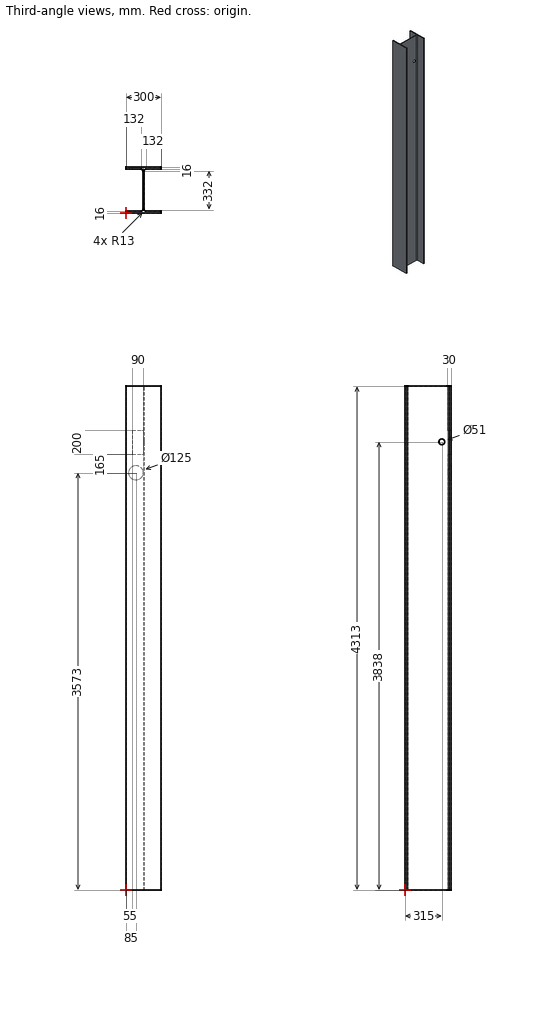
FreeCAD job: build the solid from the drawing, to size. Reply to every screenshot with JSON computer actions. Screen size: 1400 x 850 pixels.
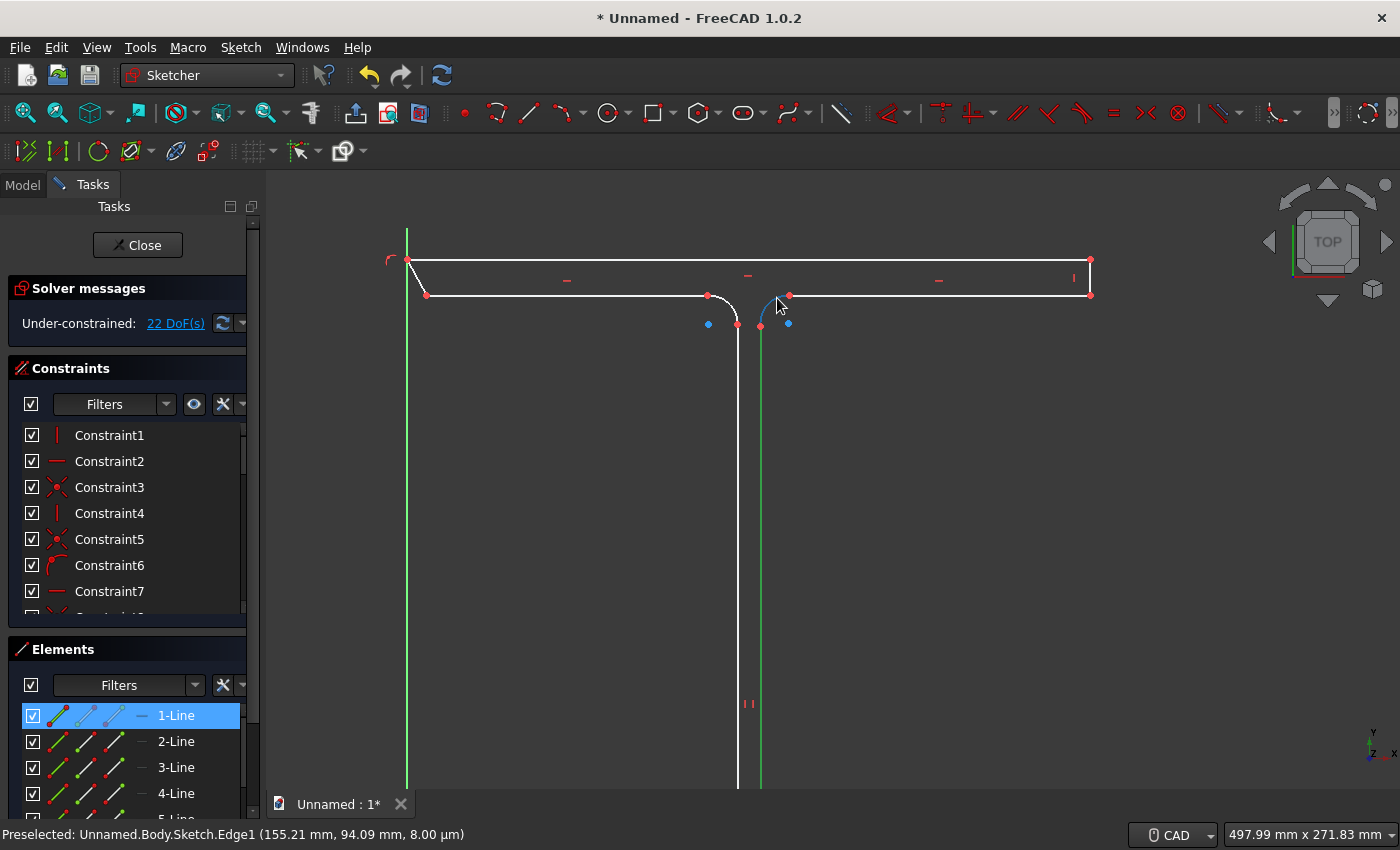
{"action": "left_click", "coordinate": [776, 299]}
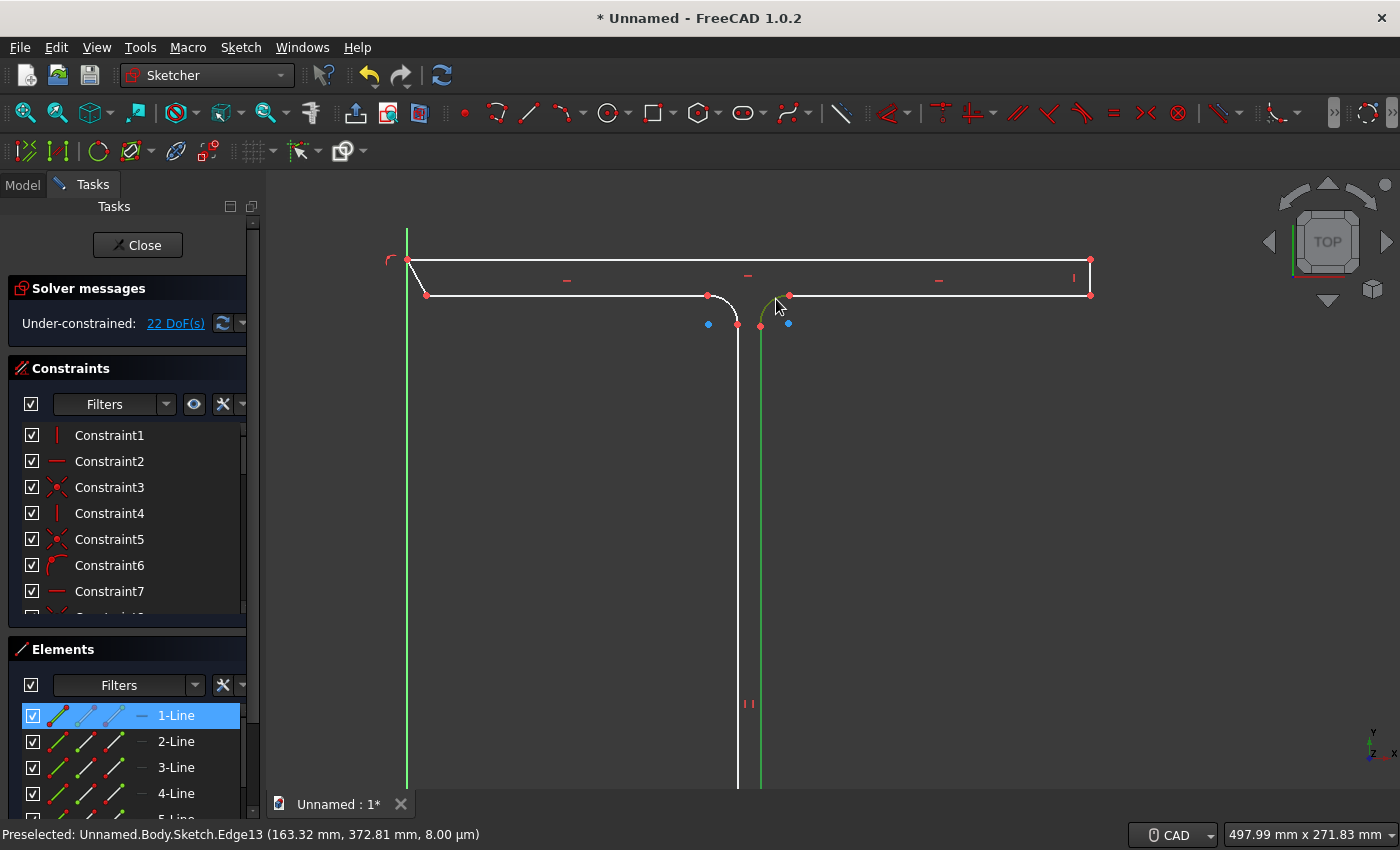
{"action": "key", "text": "t"}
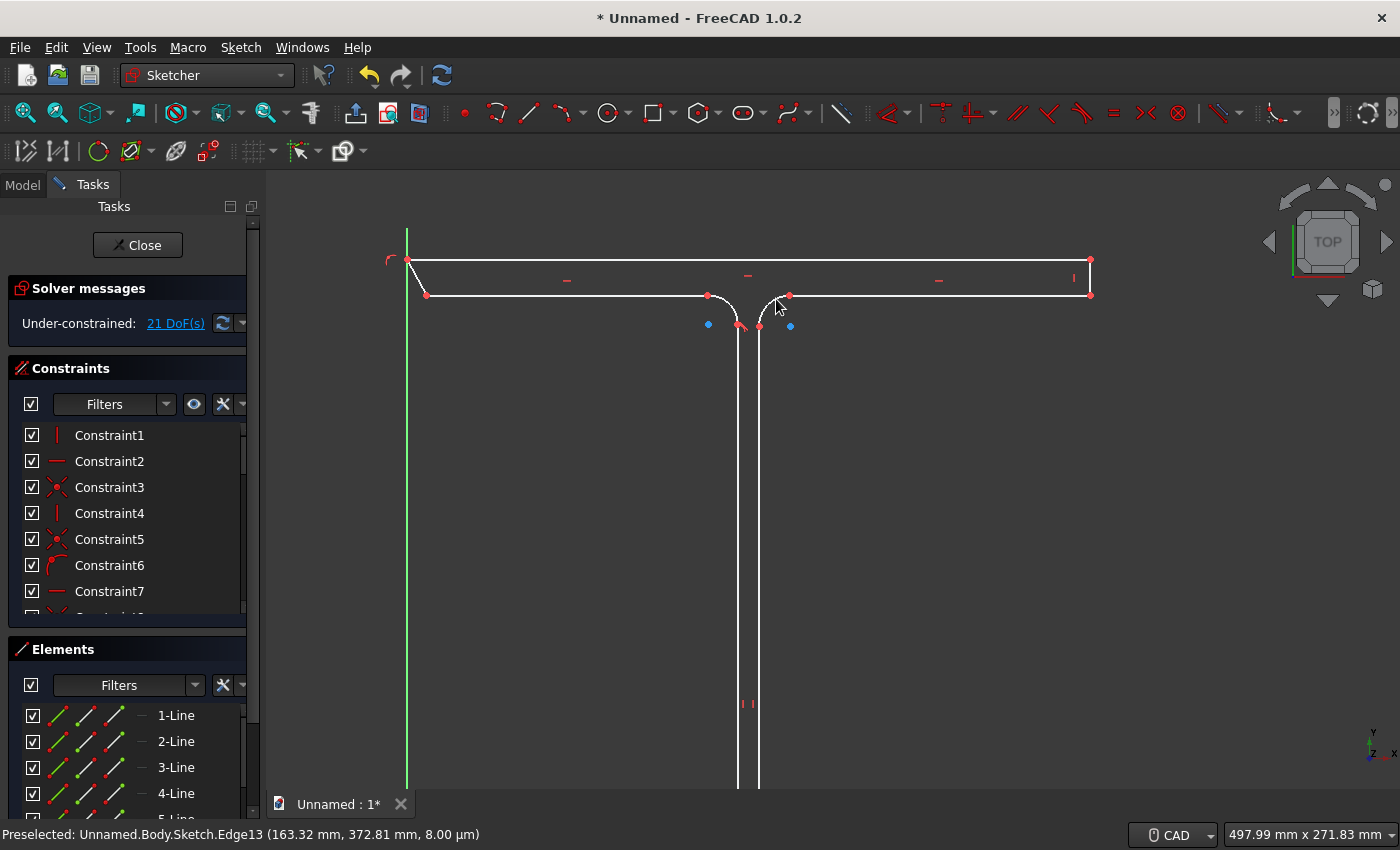
{"action": "left_click", "coordinate": [759, 553]}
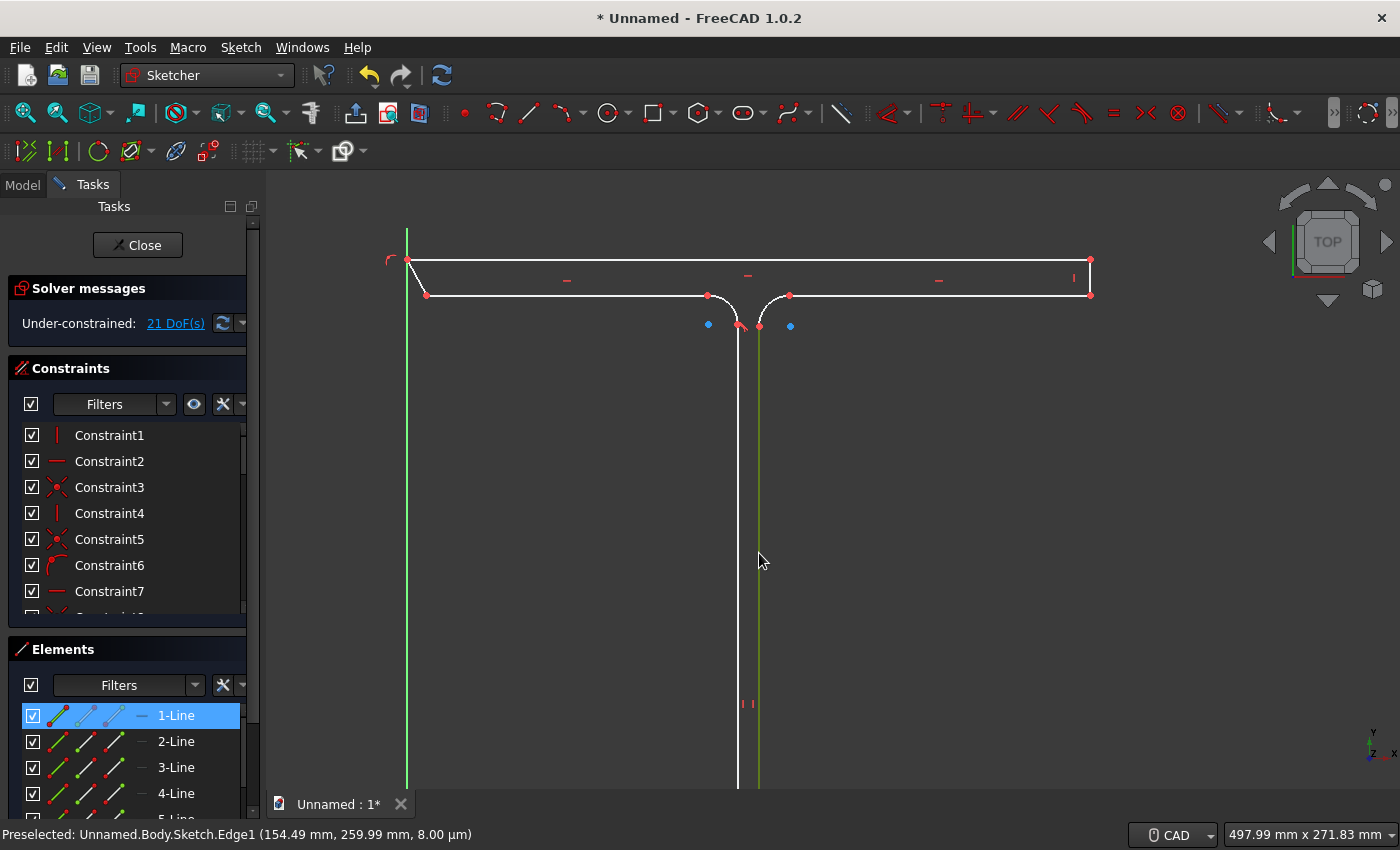
{"action": "scroll", "coordinate": [777, 298], "scroll_direction": "down", "scroll_amount": 4}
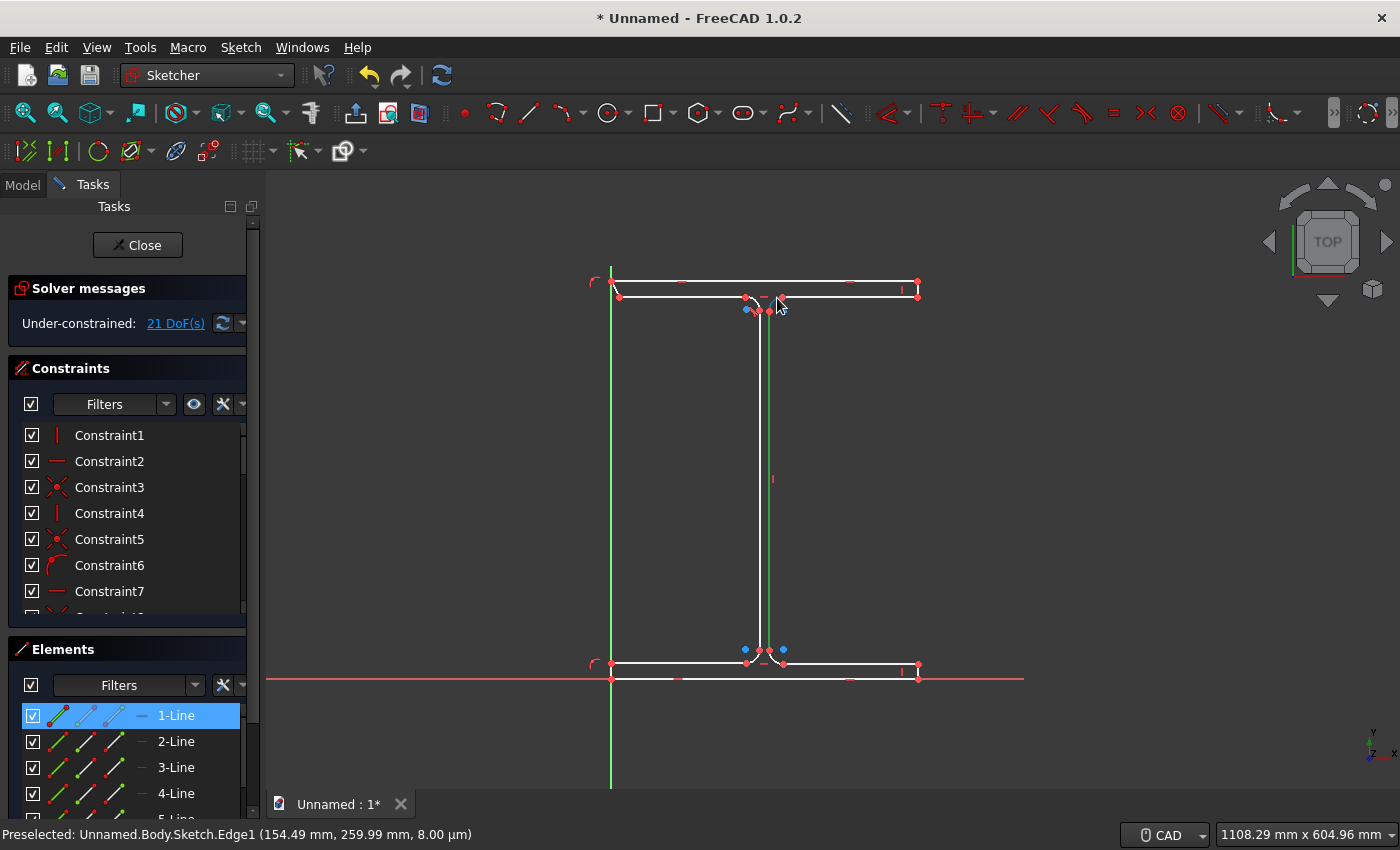
{"action": "scroll", "coordinate": [771, 656], "scroll_direction": "up", "scroll_amount": 4}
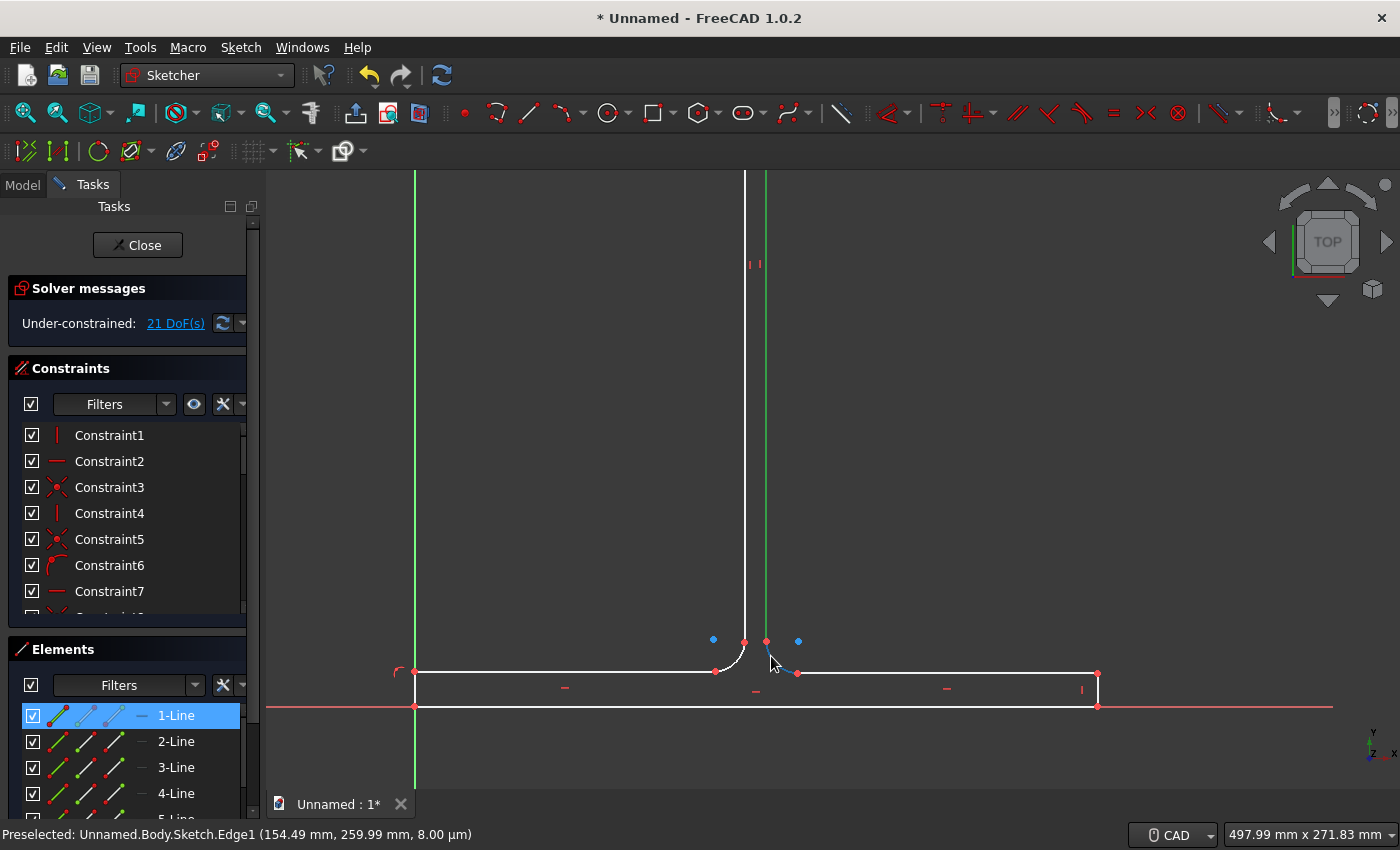
{"action": "left_click", "coordinate": [770, 656]}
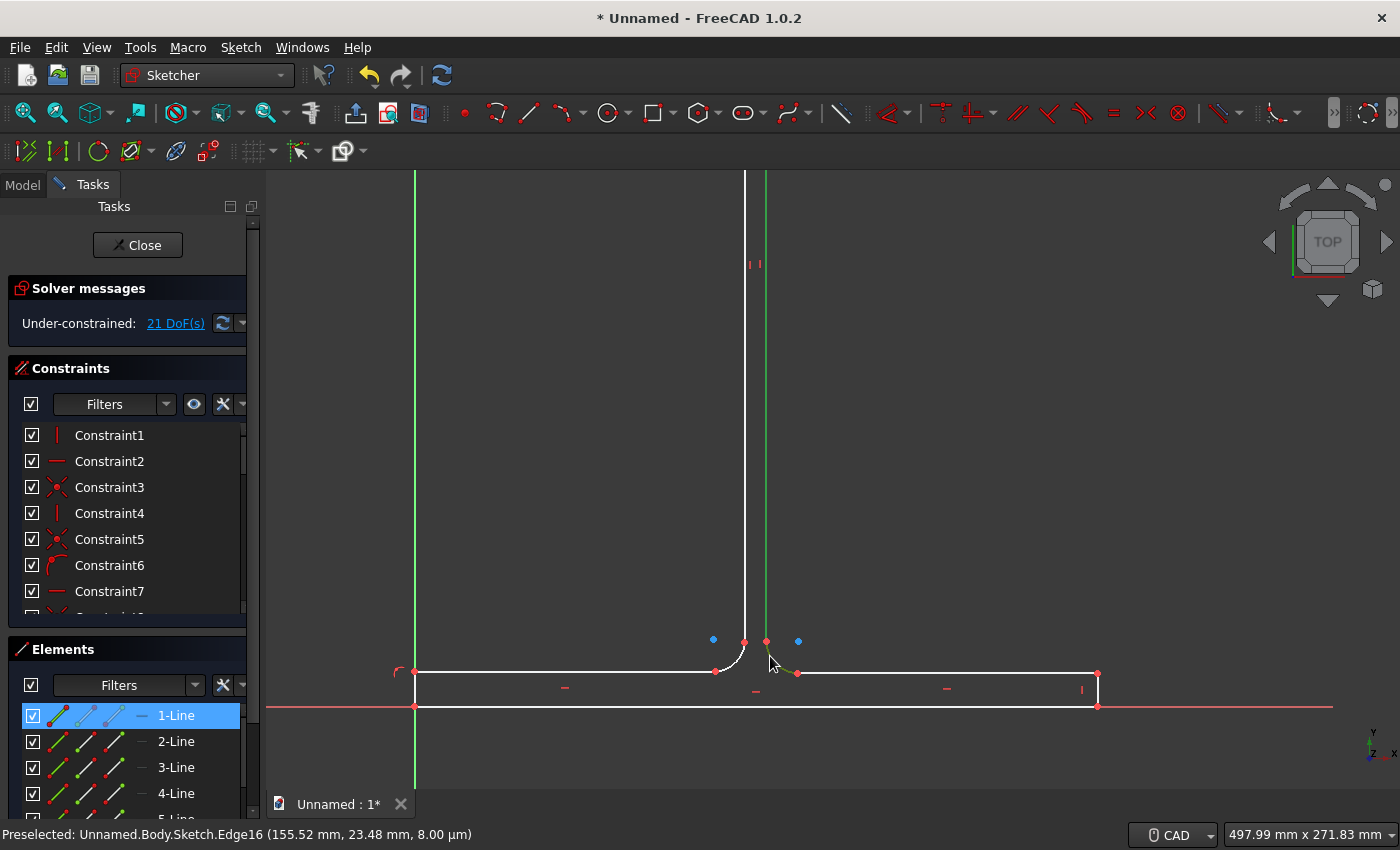
{"action": "left_click", "coordinate": [1082, 114]}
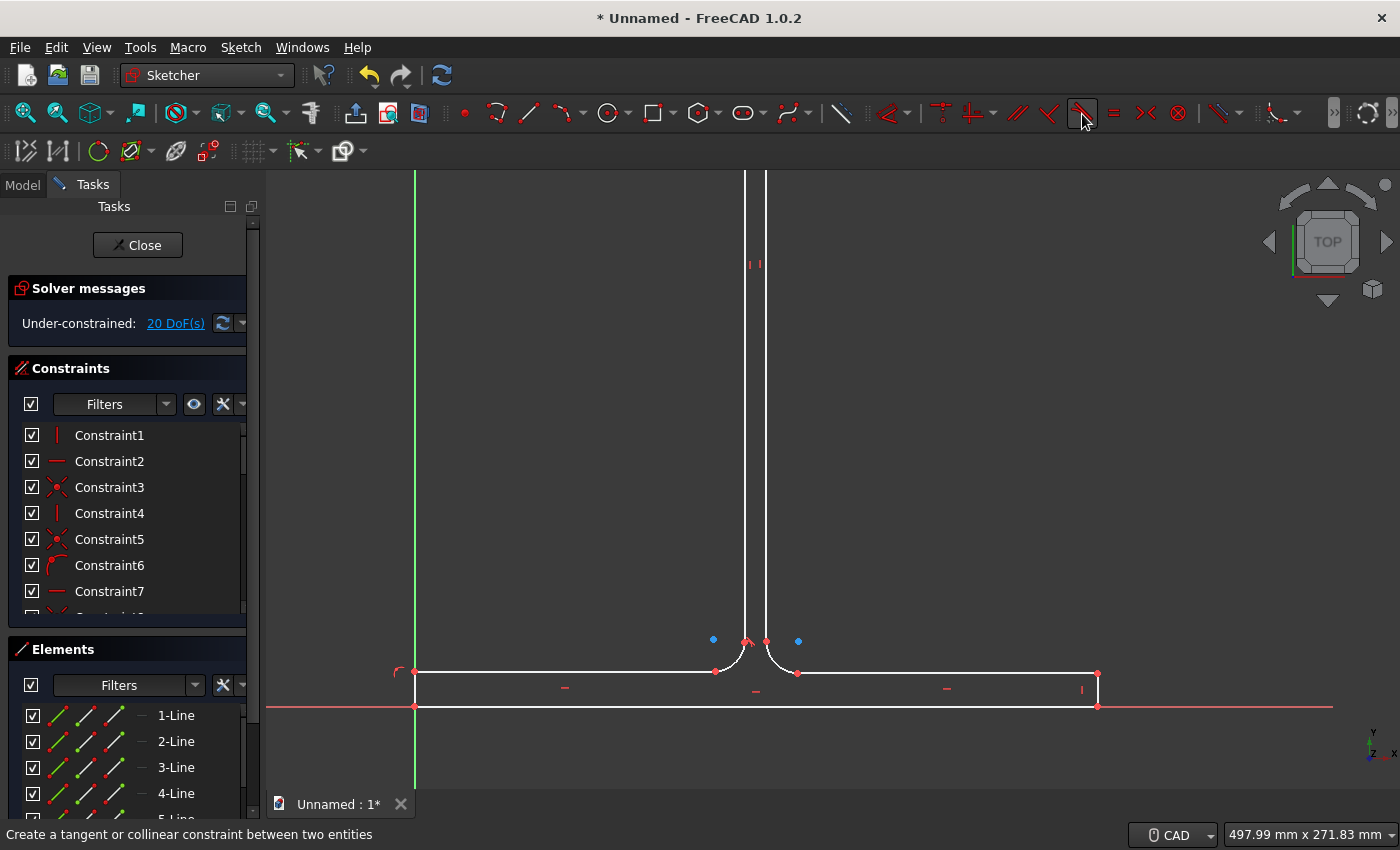
{"action": "scroll", "coordinate": [771, 657], "scroll_direction": "down", "scroll_amount": 4}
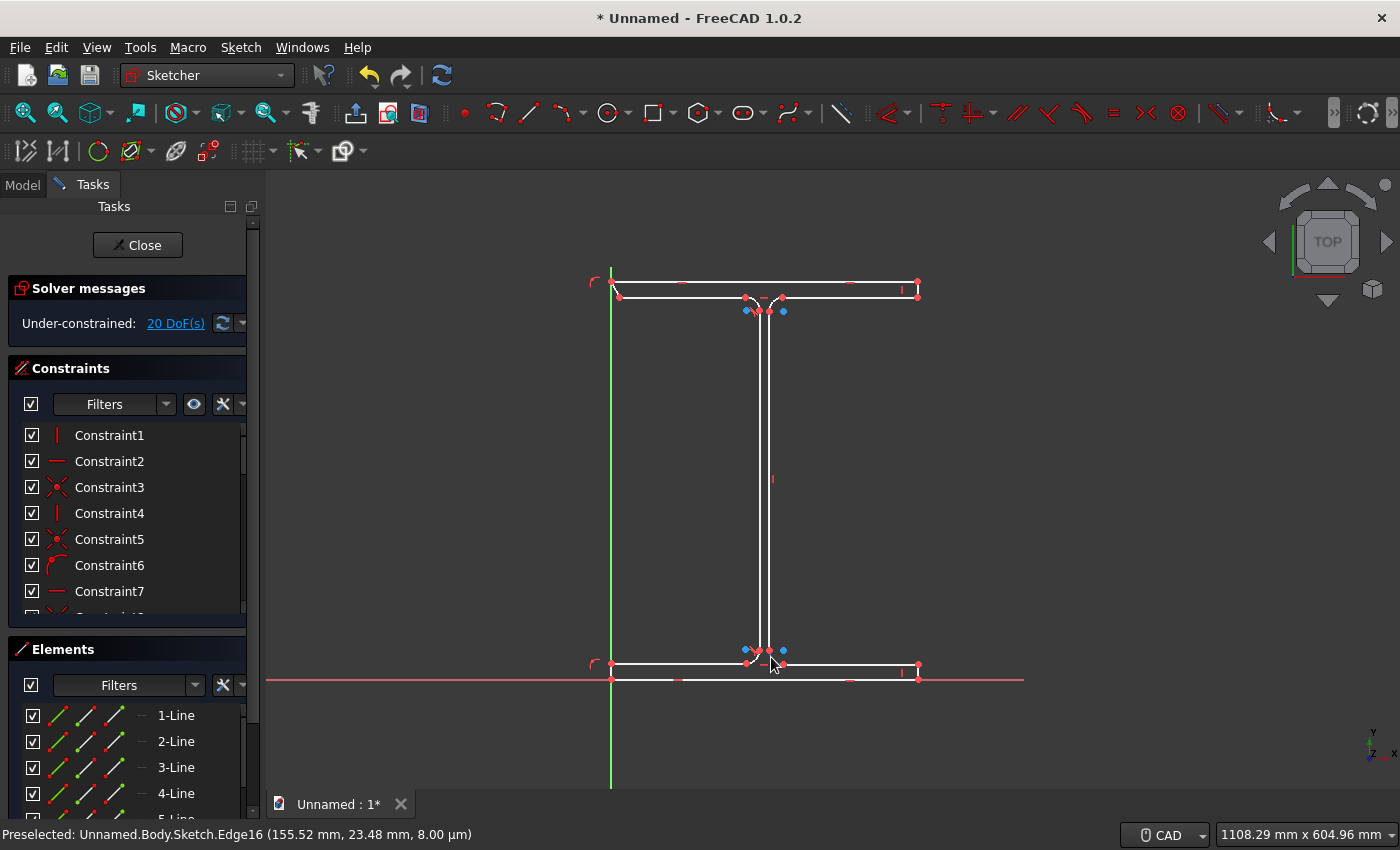
{"action": "left_click", "coordinate": [823, 298]}